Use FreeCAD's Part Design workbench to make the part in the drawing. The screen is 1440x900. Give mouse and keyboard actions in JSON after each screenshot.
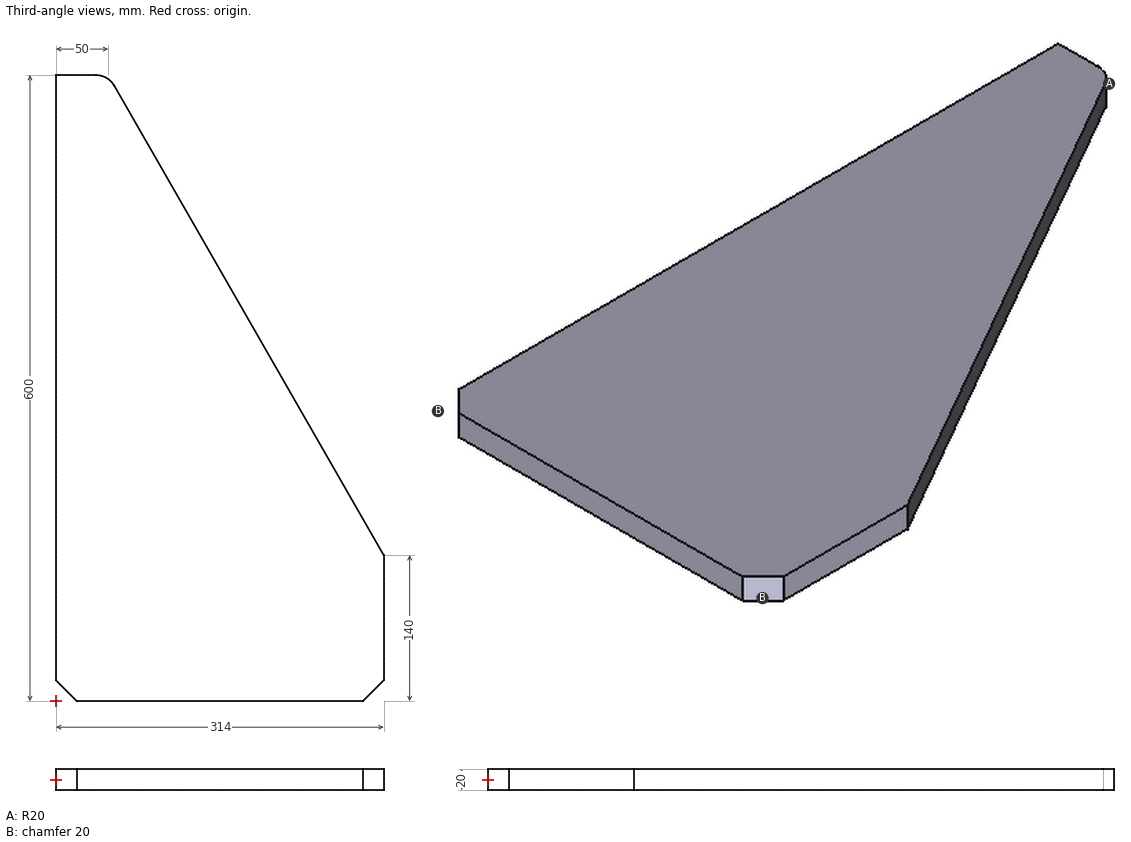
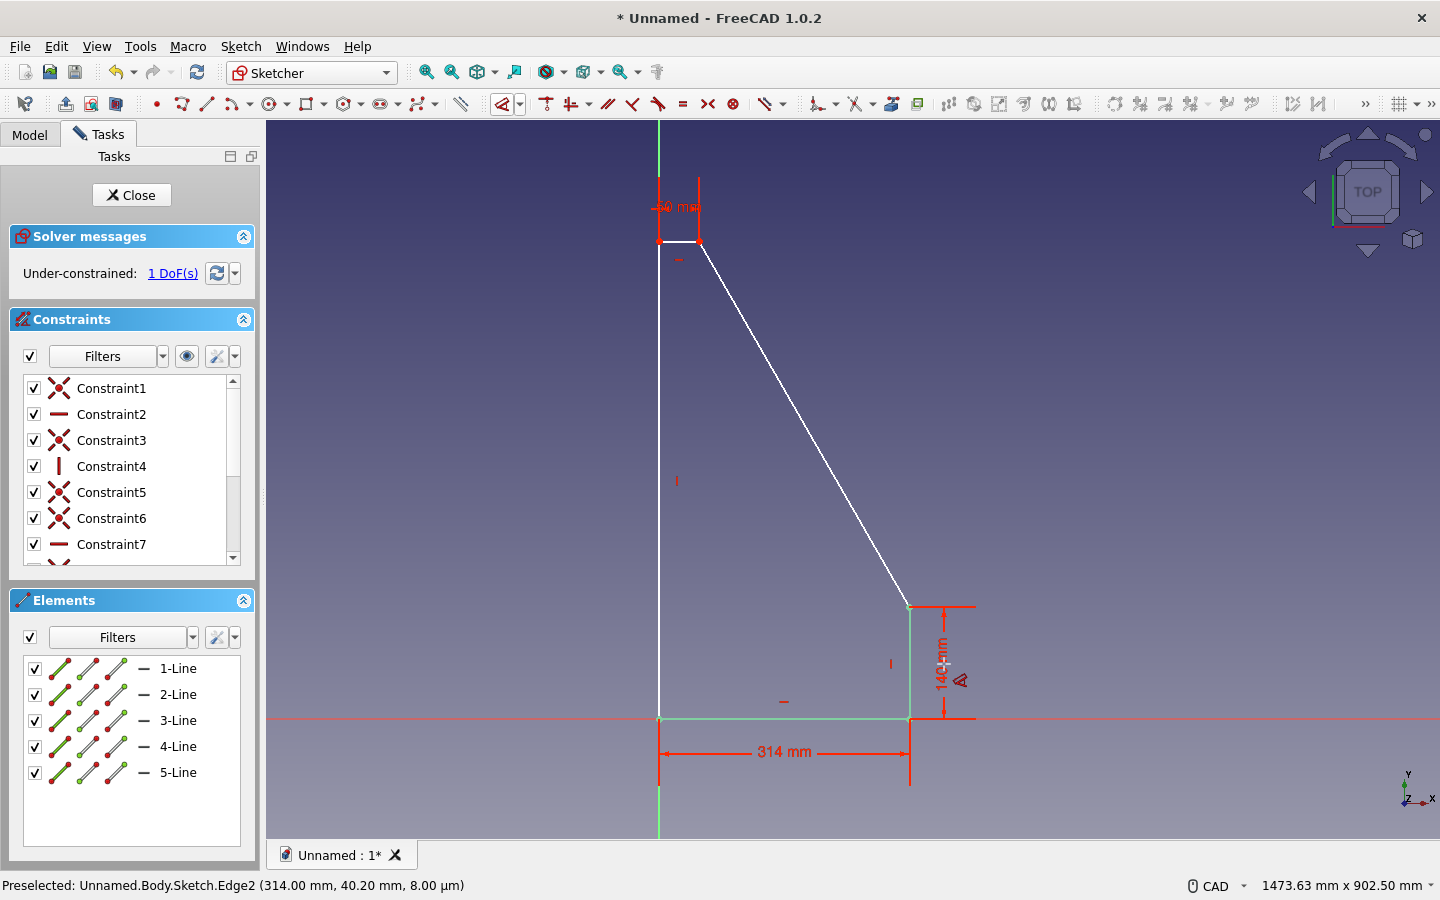
{"action": "left_click", "coordinate": [659, 385]}
{"action": "left_click", "coordinate": [625, 481]}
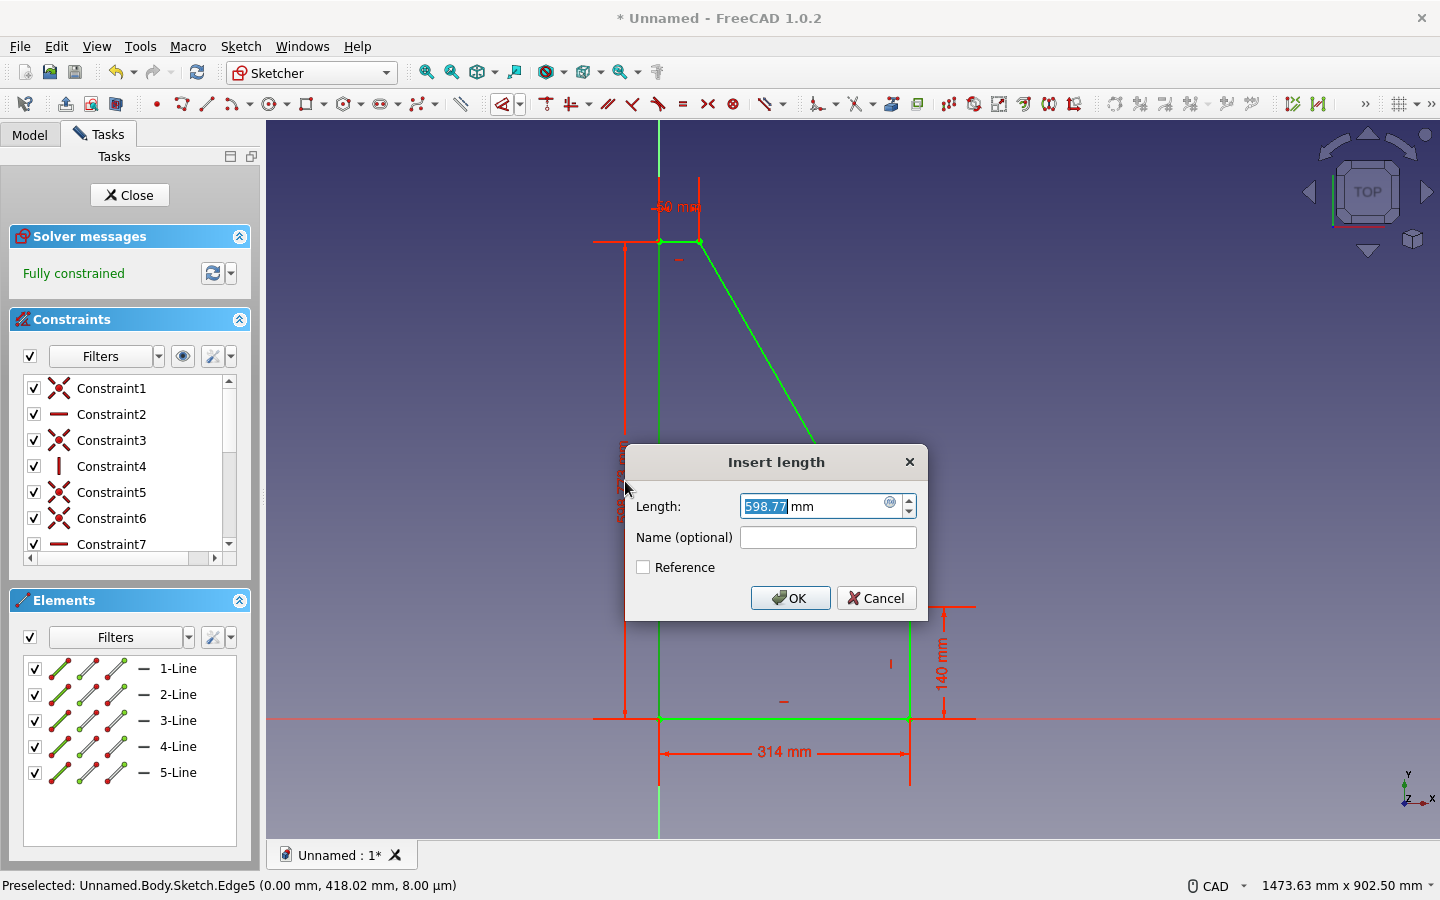
{"action": "type", "text": "600"}
{"action": "key", "text": "Return"}
{"action": "key", "text": "Escape"}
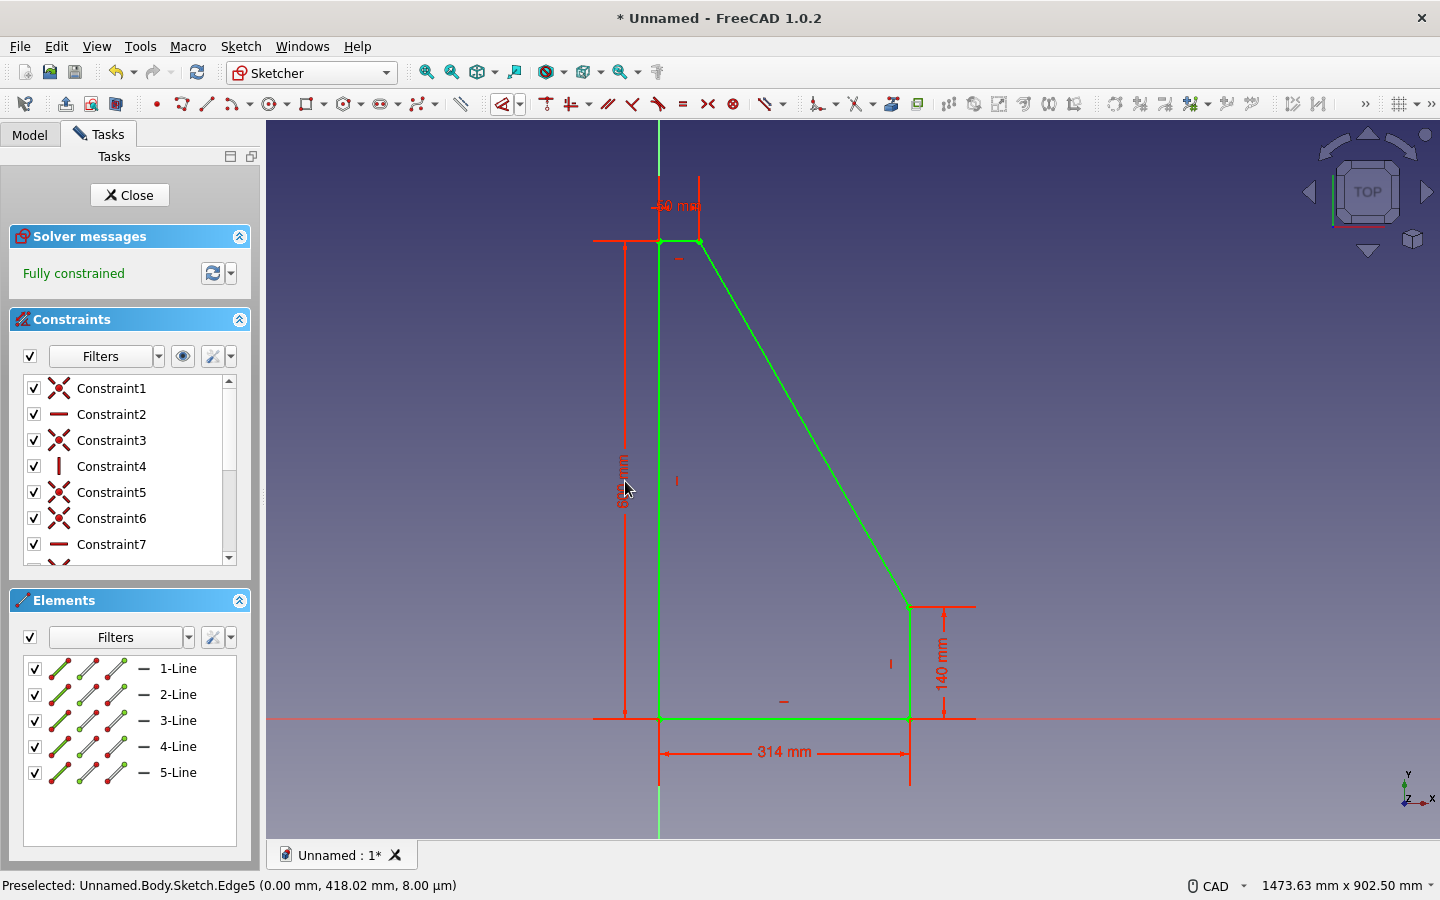
{"action": "left_click", "coordinate": [130, 195]}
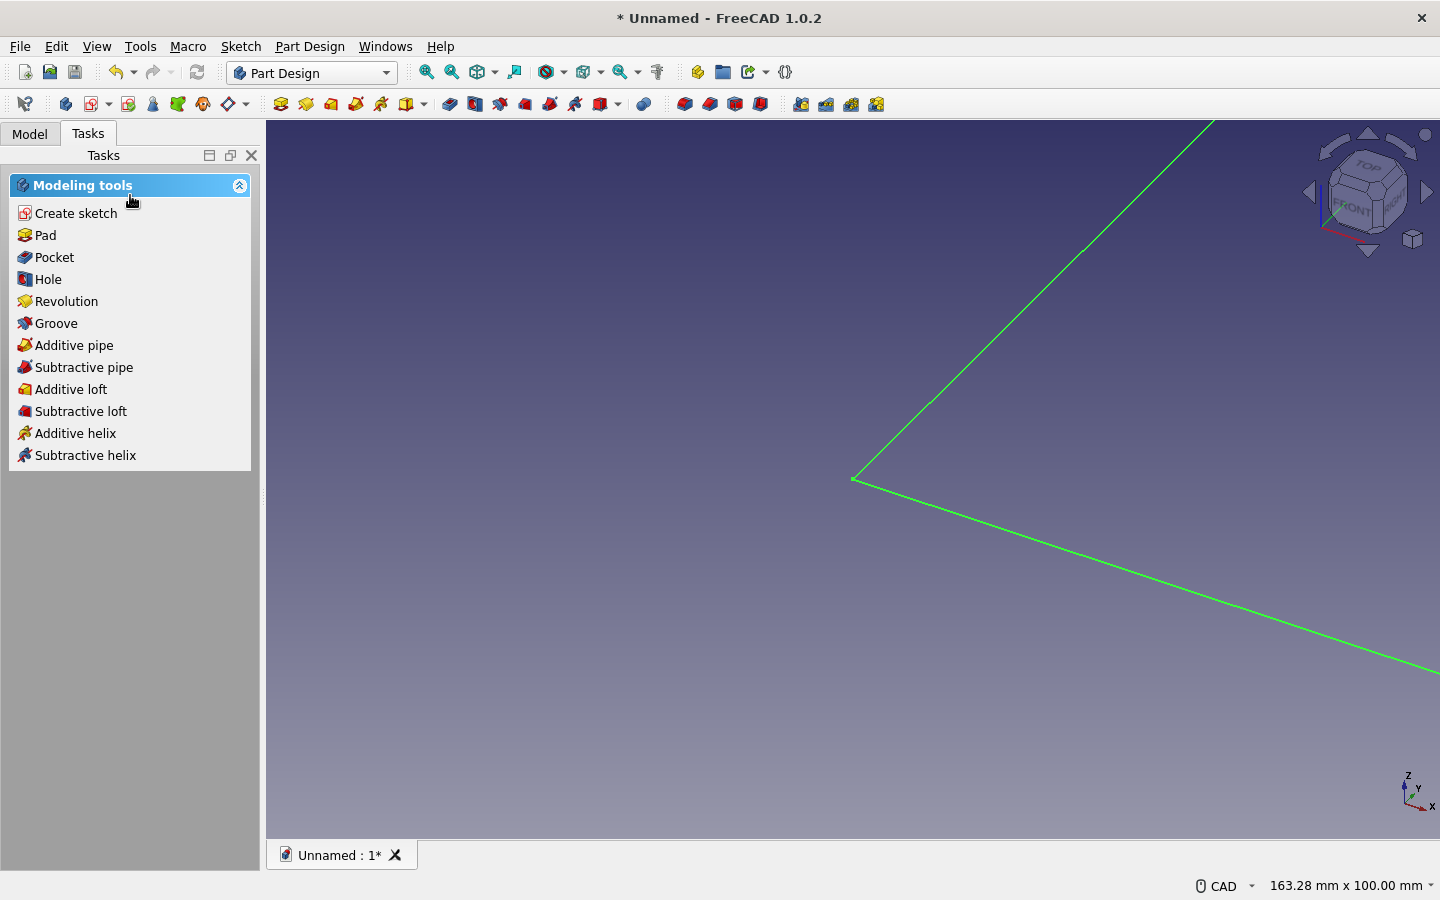
{"action": "left_click", "coordinate": [281, 104]}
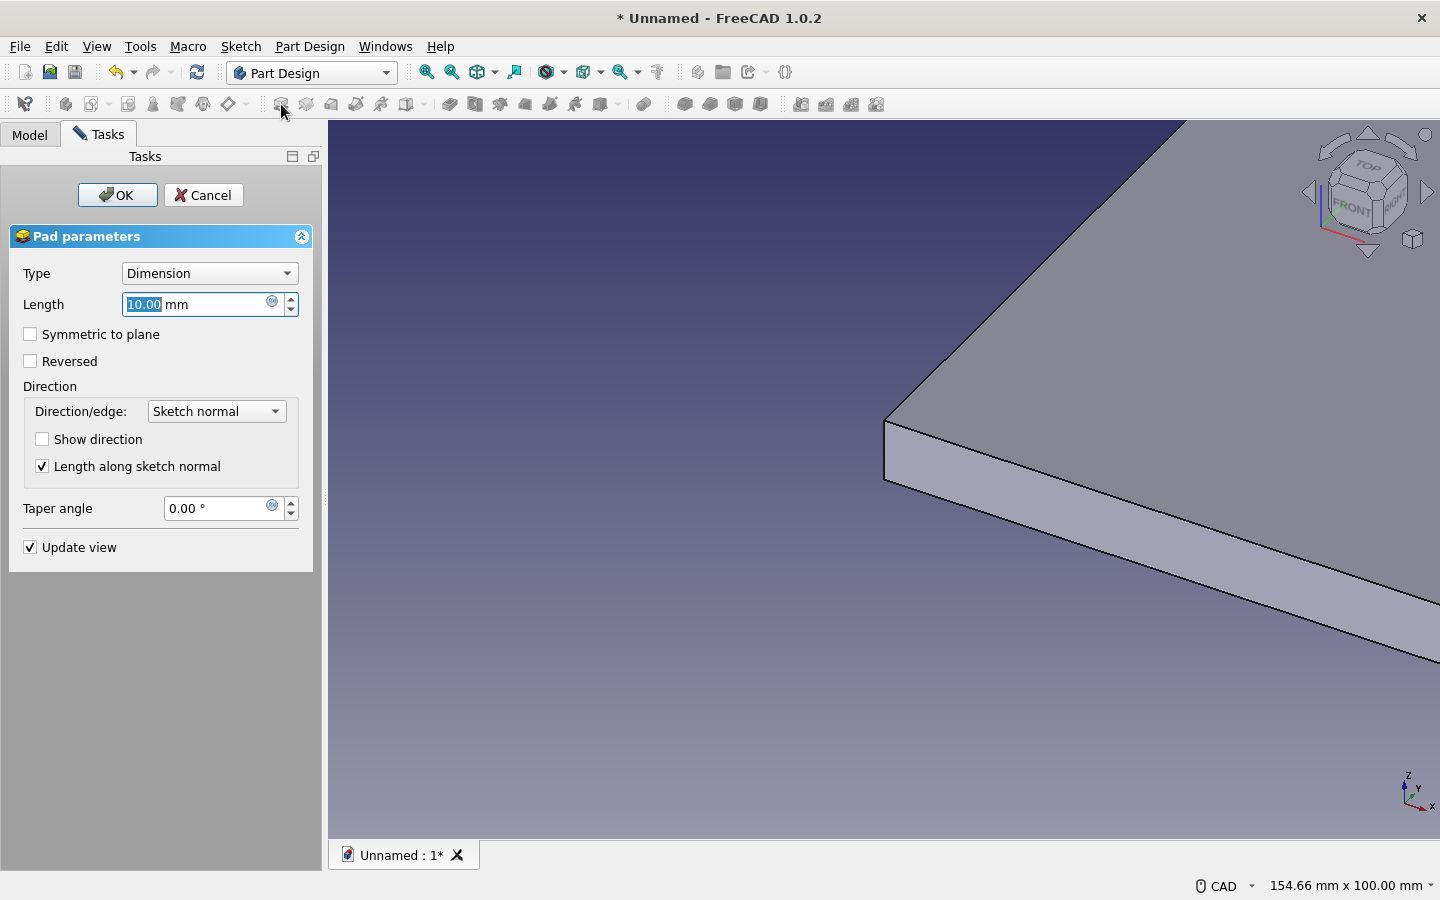
{"action": "type", "text": "20"}
{"action": "key", "text": "Tab"}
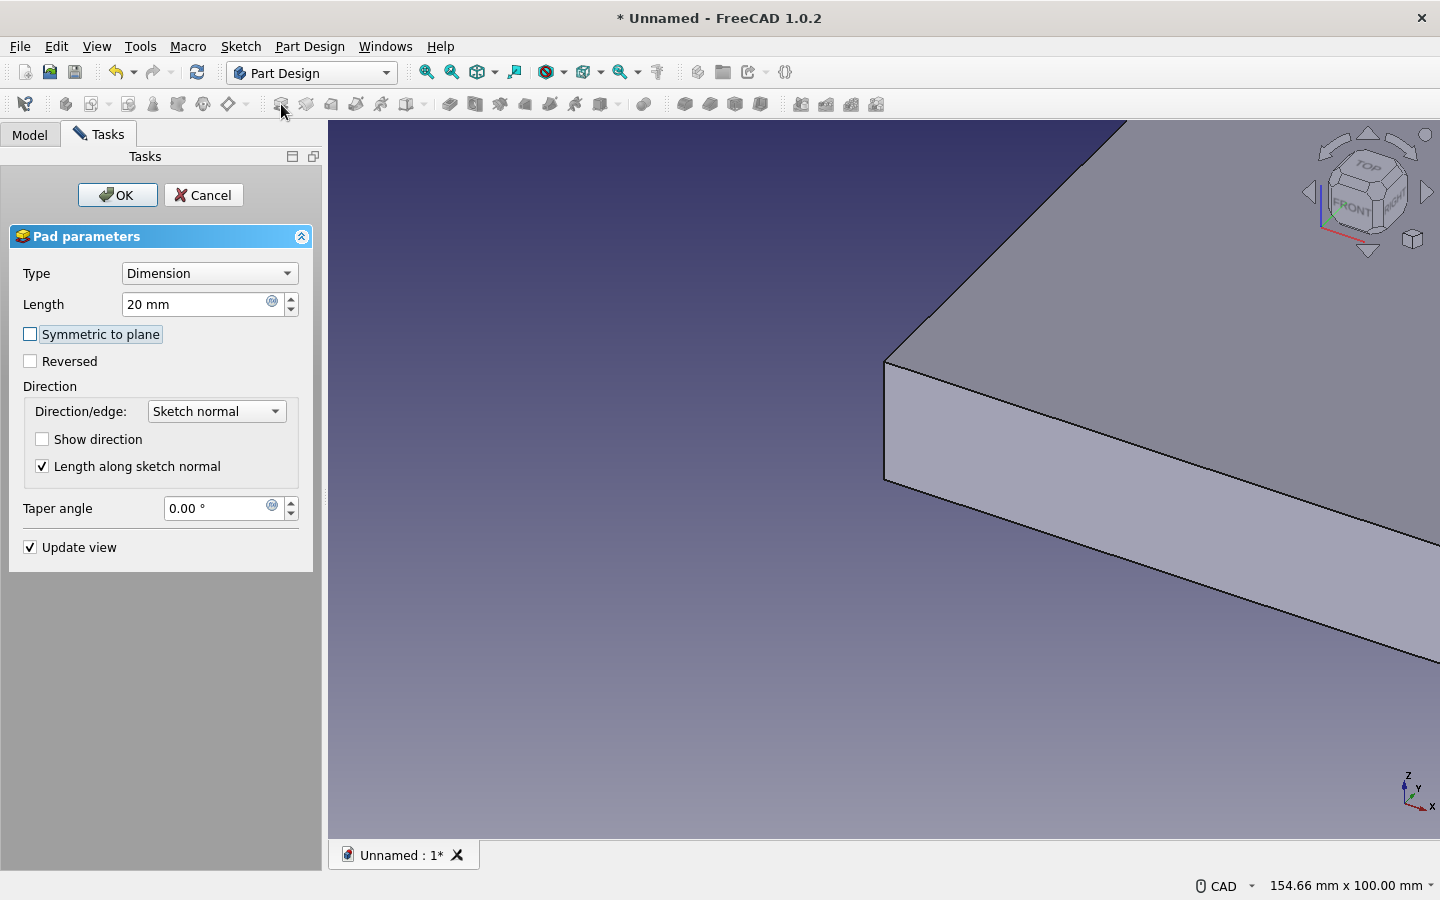
{"action": "left_click", "coordinate": [31, 334]}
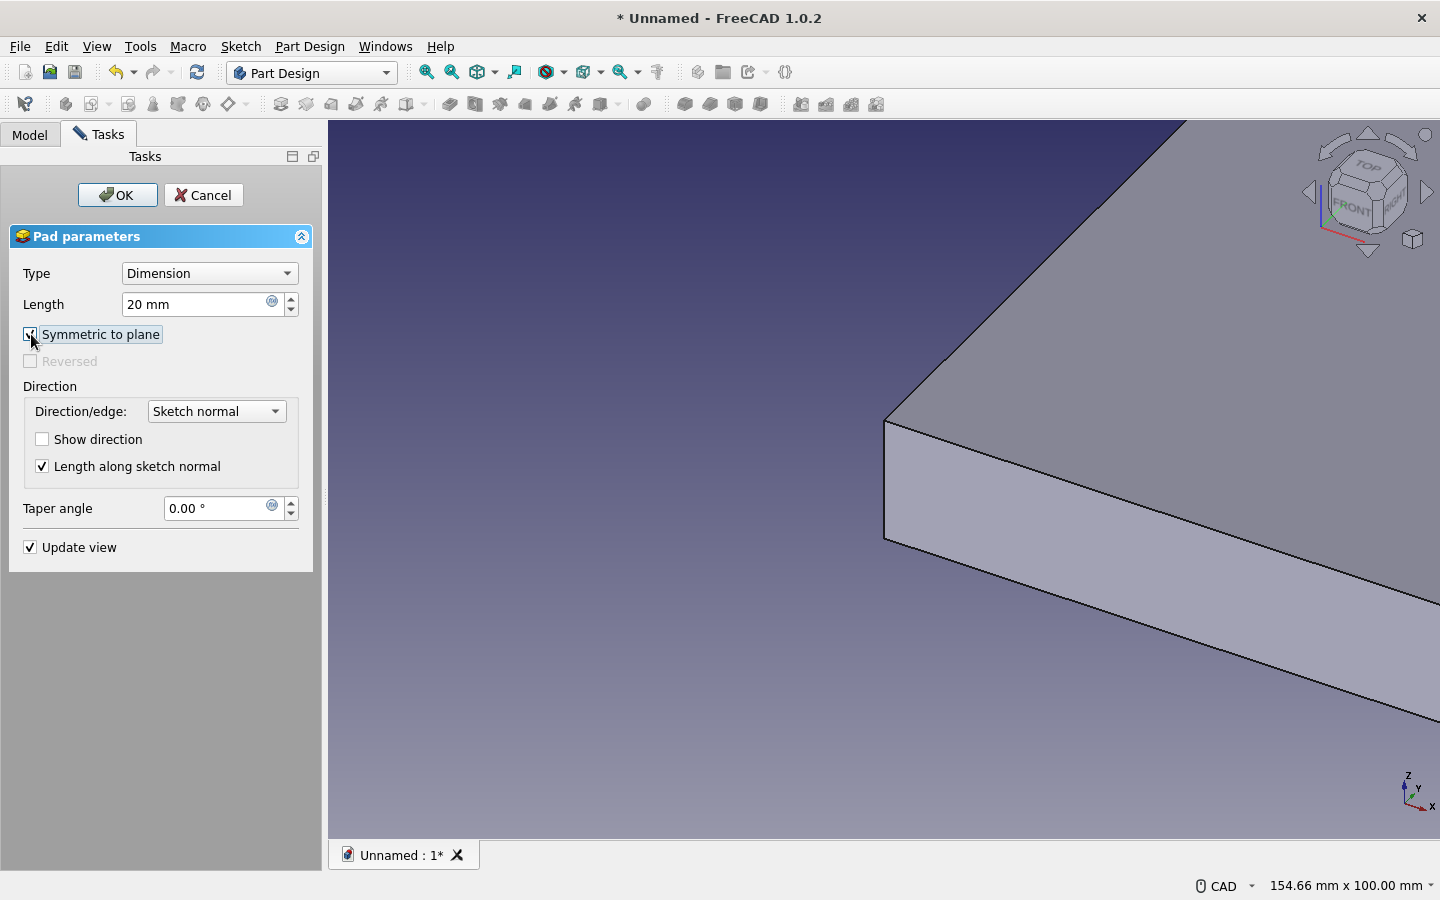
{"action": "left_click", "coordinate": [118, 195]}